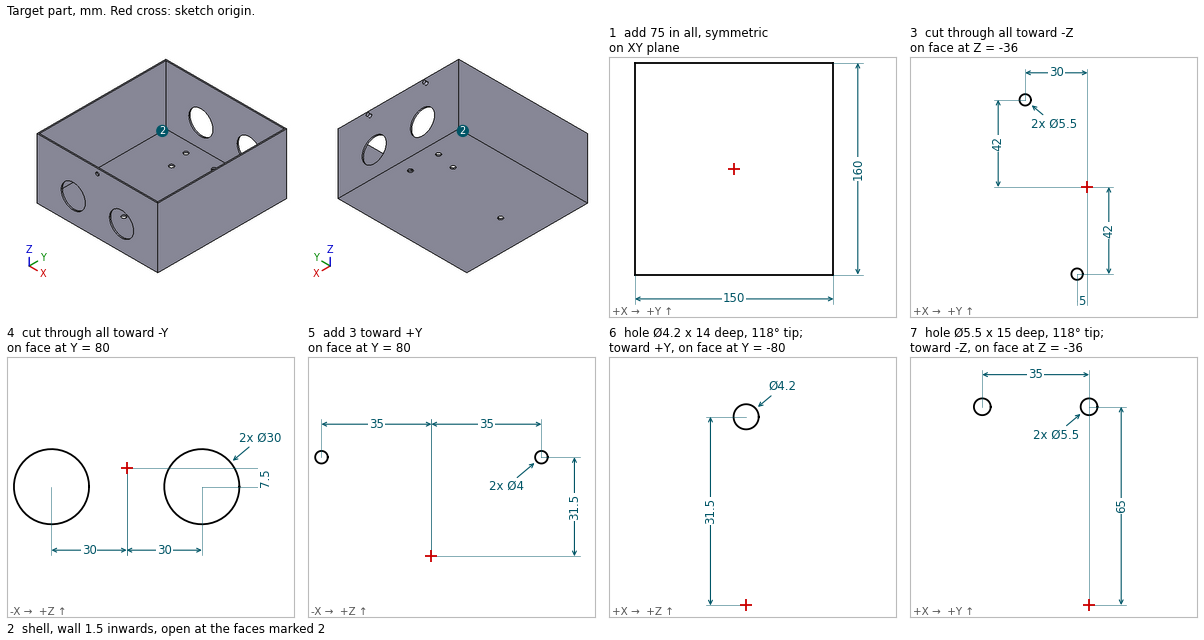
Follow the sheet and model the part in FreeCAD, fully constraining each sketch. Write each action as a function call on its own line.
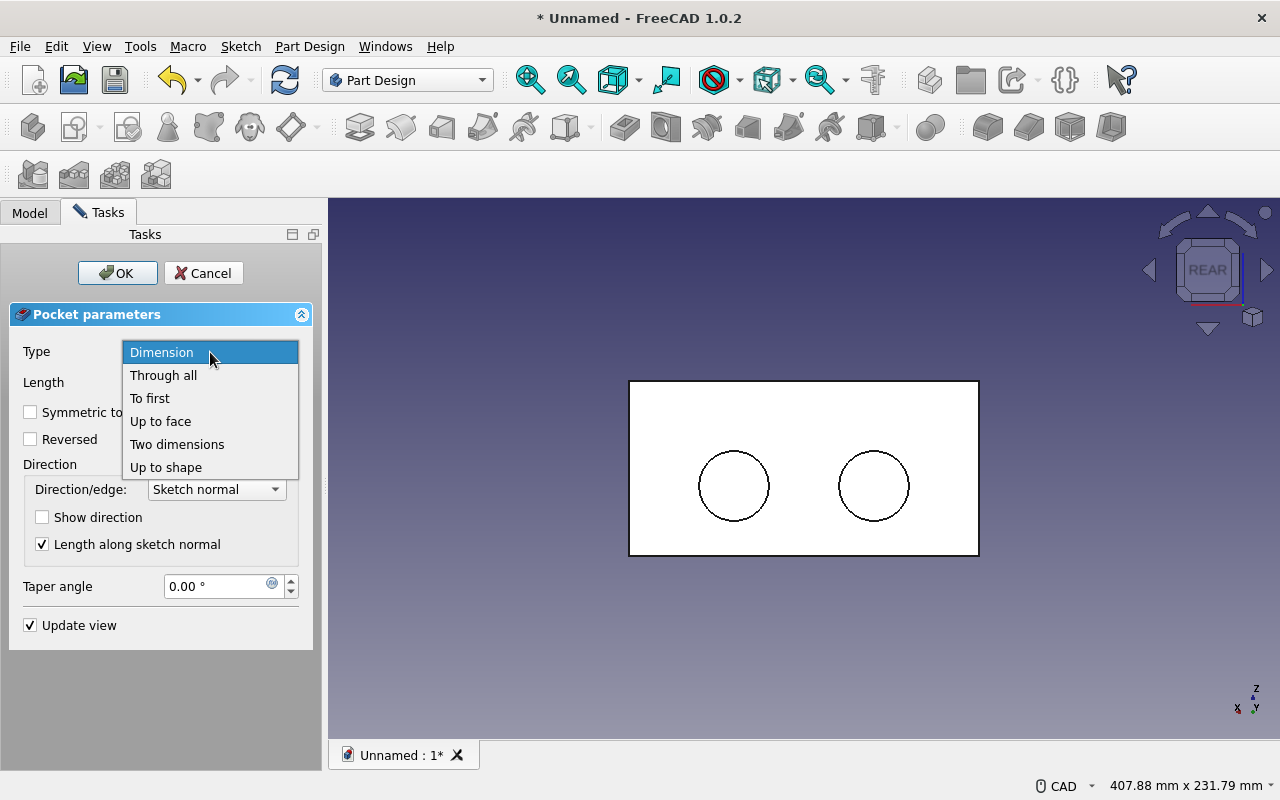
click(208, 376)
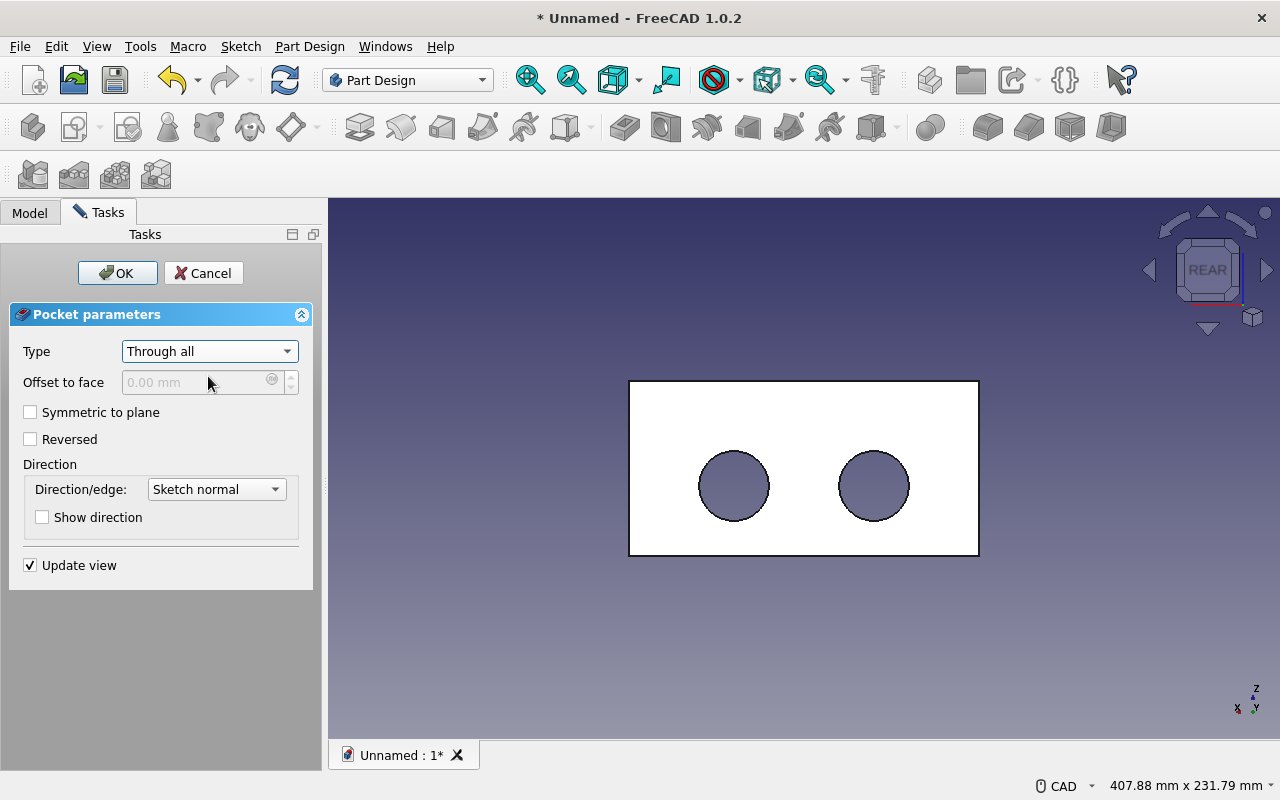
click(118, 273)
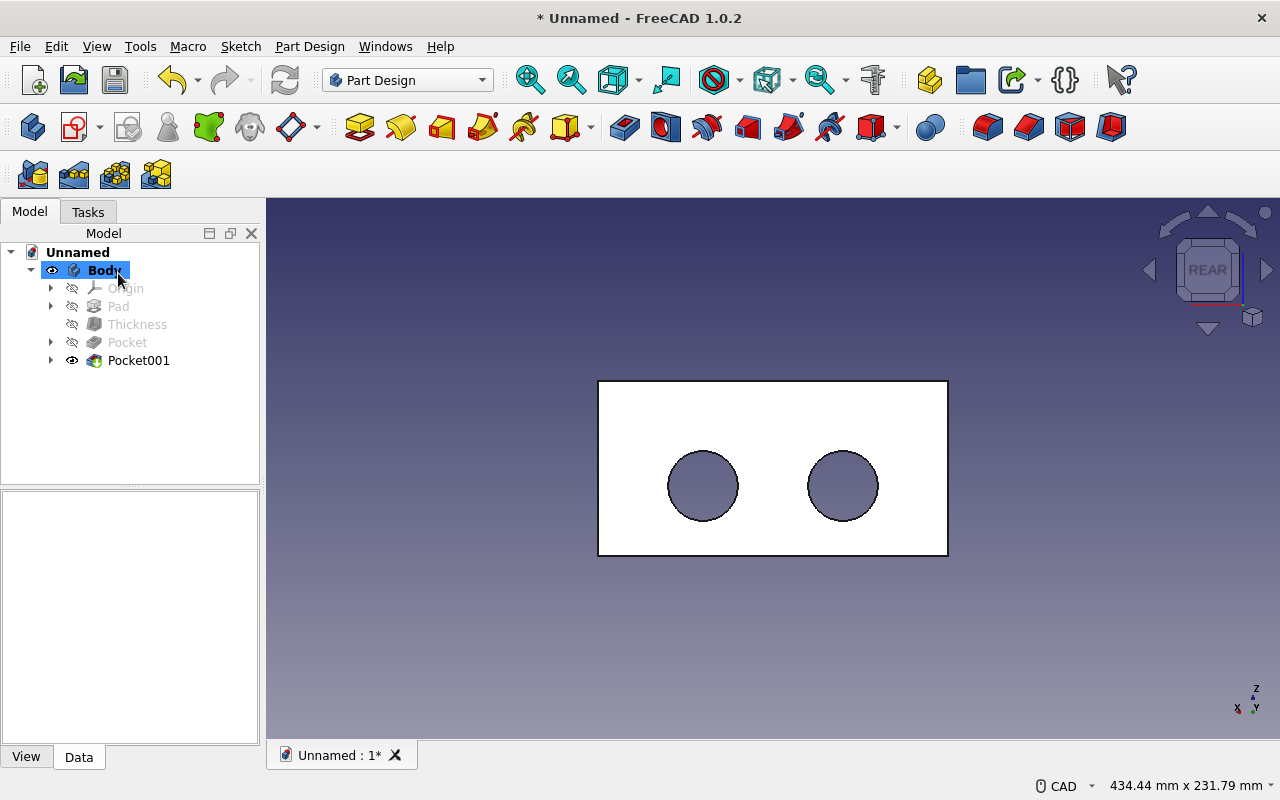
key(v)
key(f)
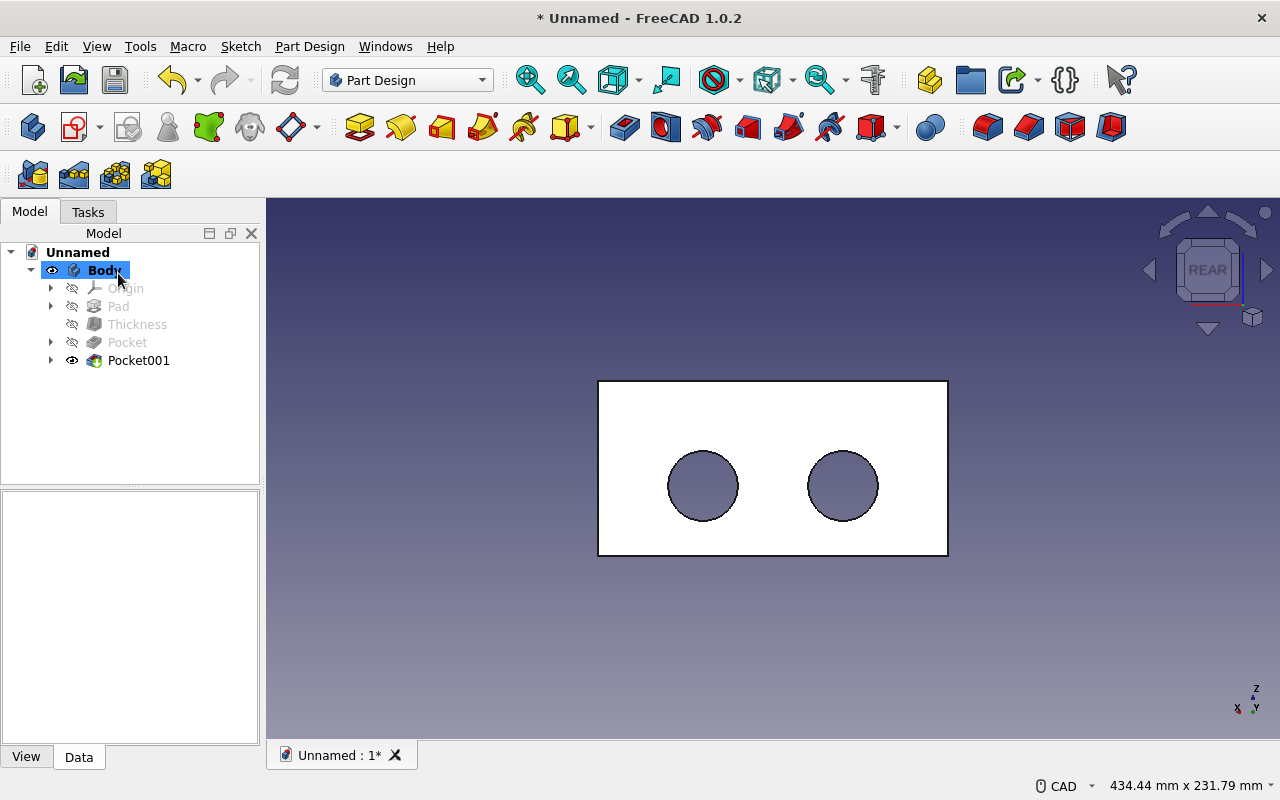
click(773, 442)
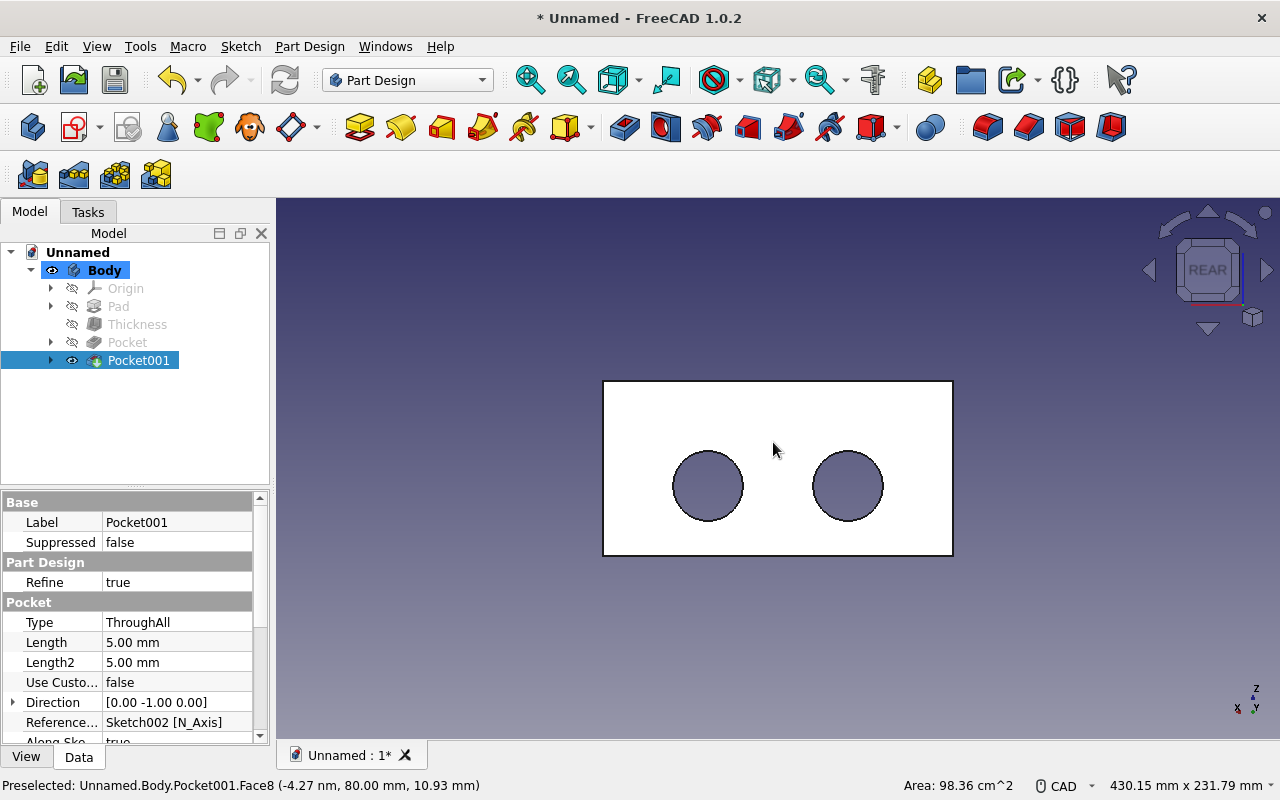
click(74, 128)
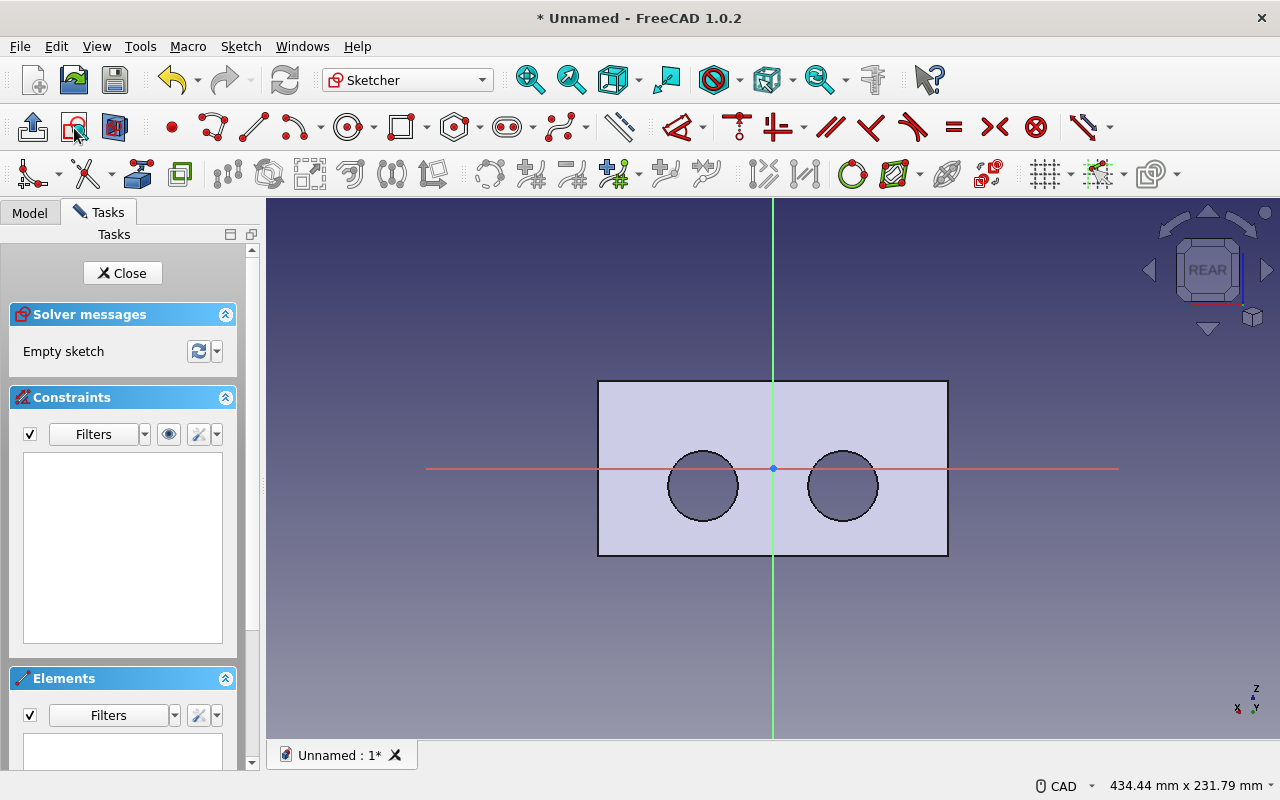
scroll(803, 413, up, 6)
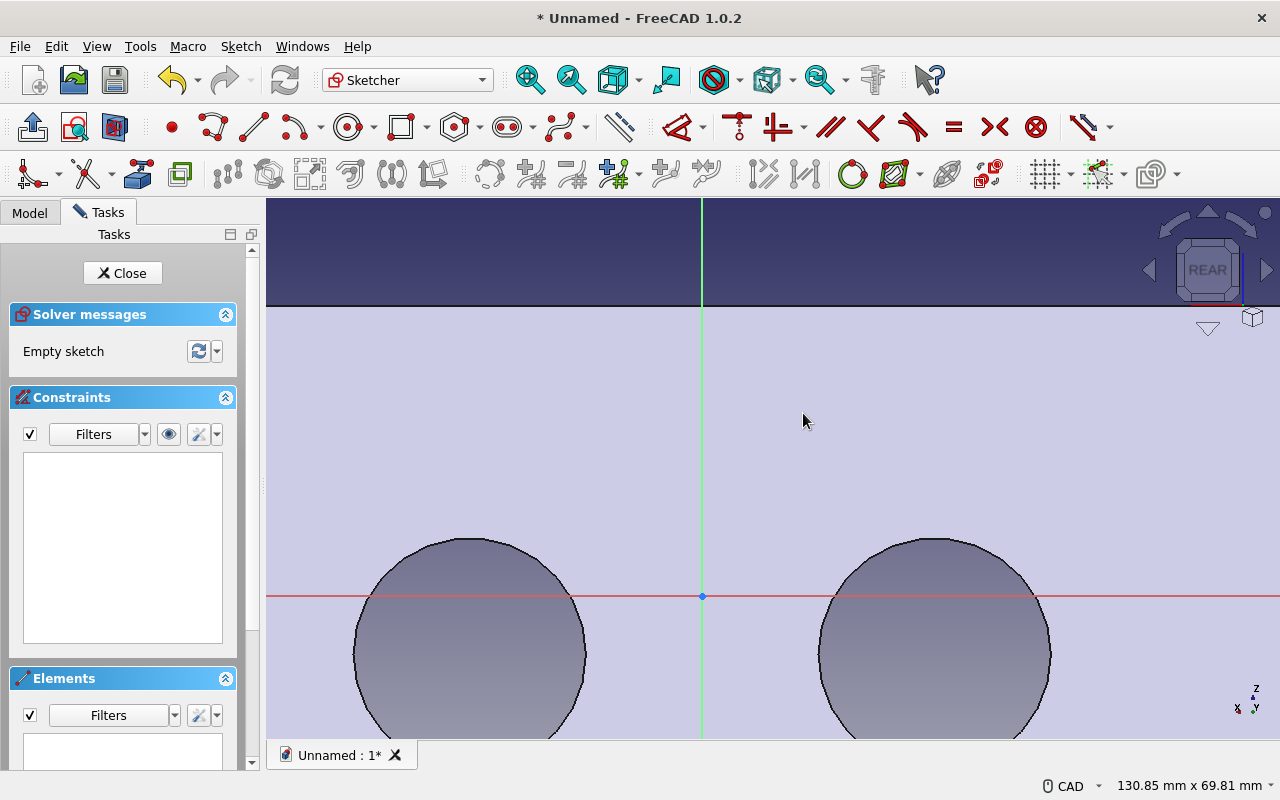
key(g)
key(c)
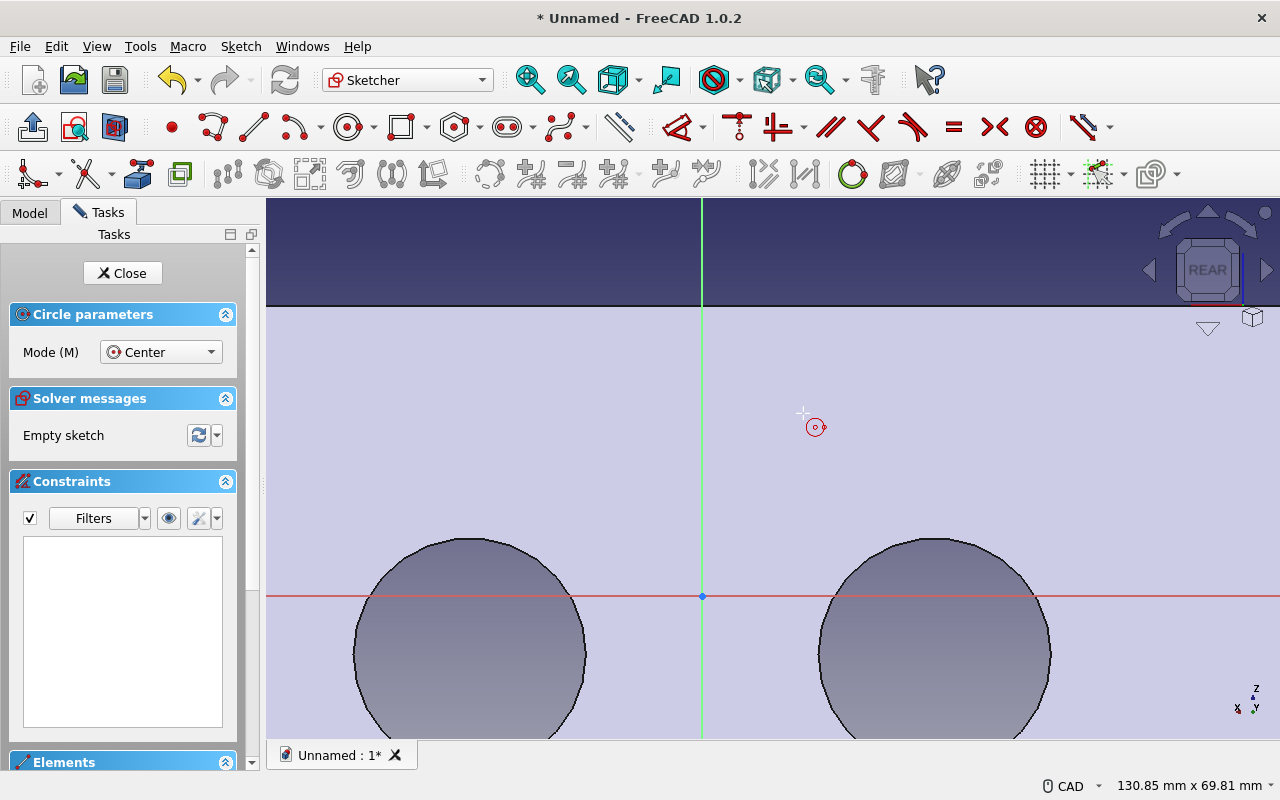
scroll(973, 352, up, 2)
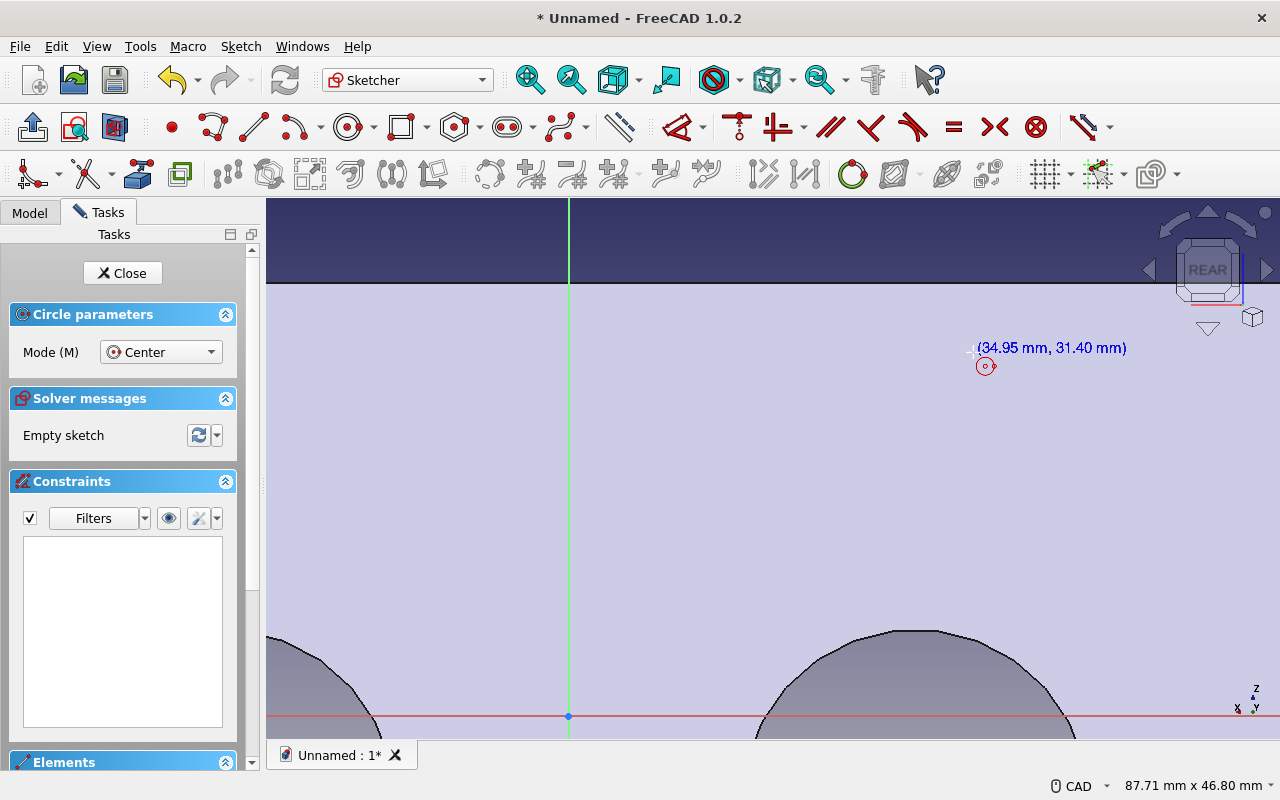
click(973, 352)
move(990, 336)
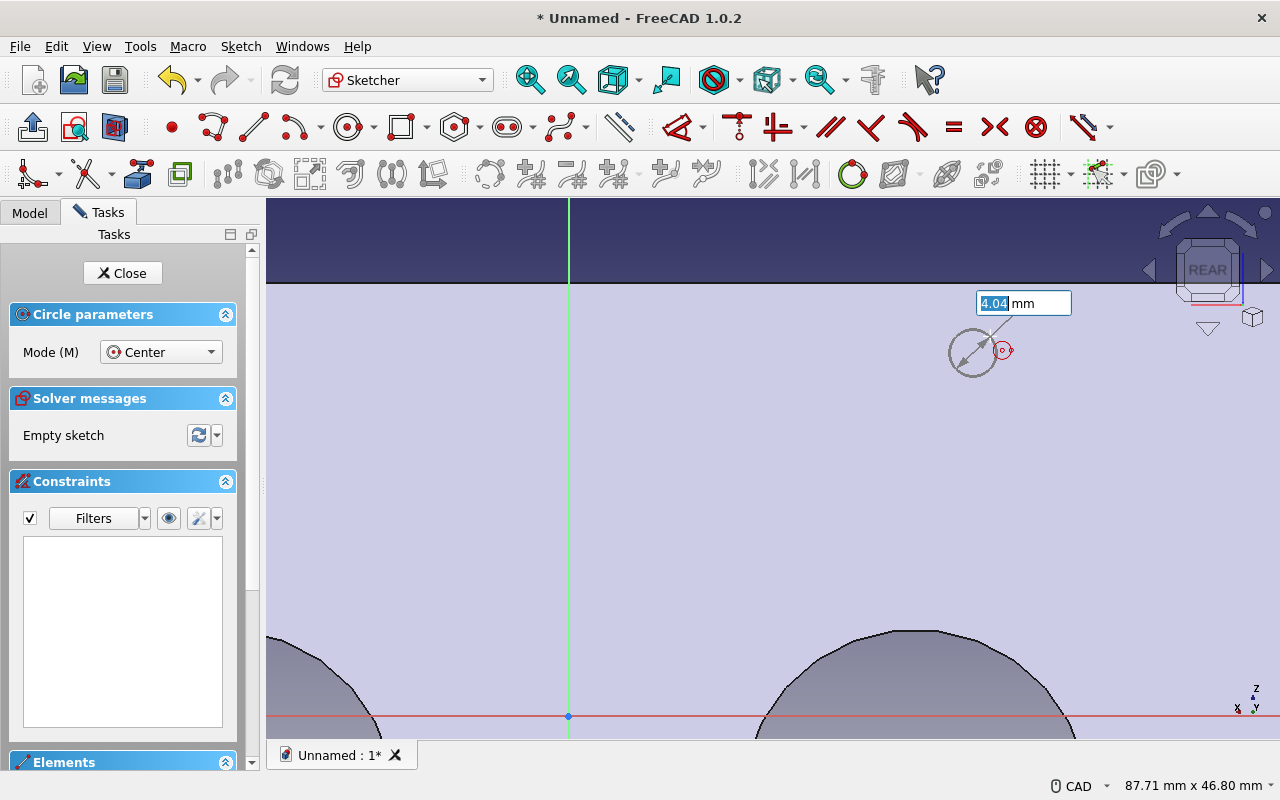
text(4)
key(Return)